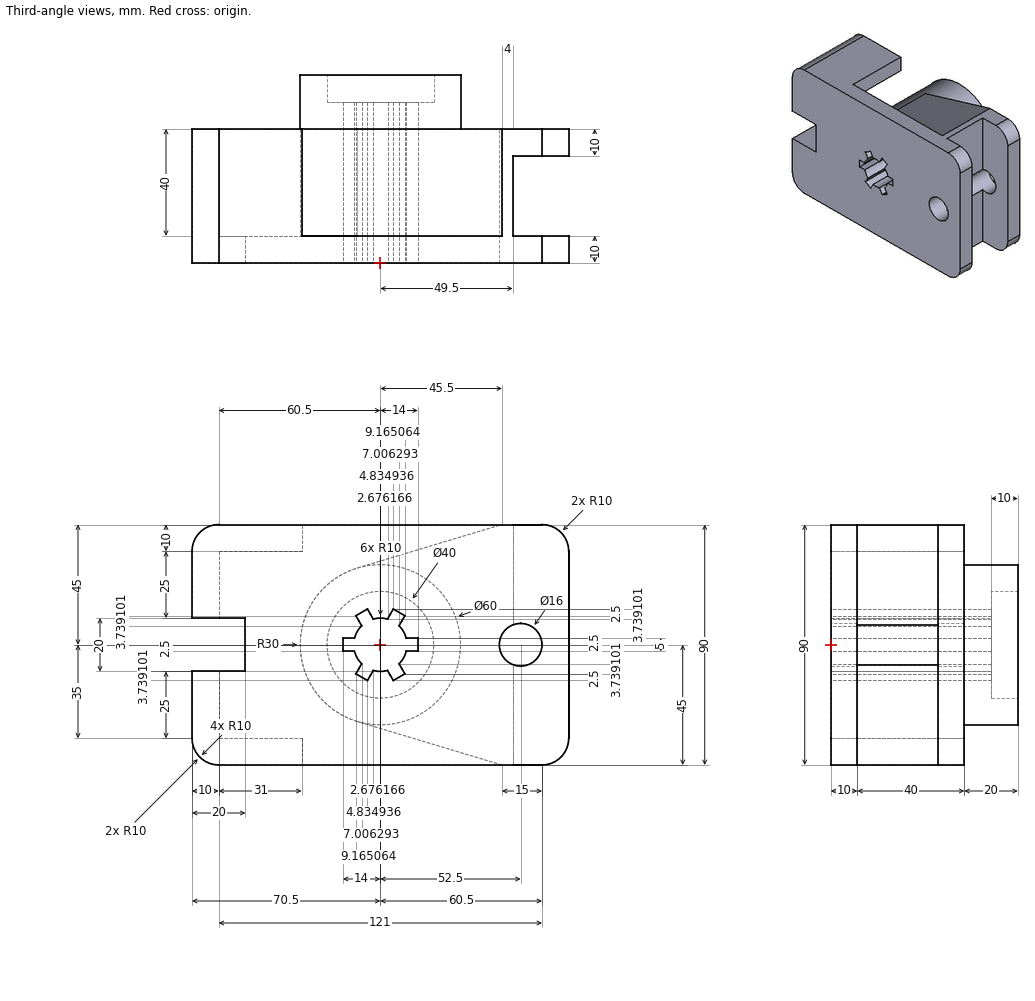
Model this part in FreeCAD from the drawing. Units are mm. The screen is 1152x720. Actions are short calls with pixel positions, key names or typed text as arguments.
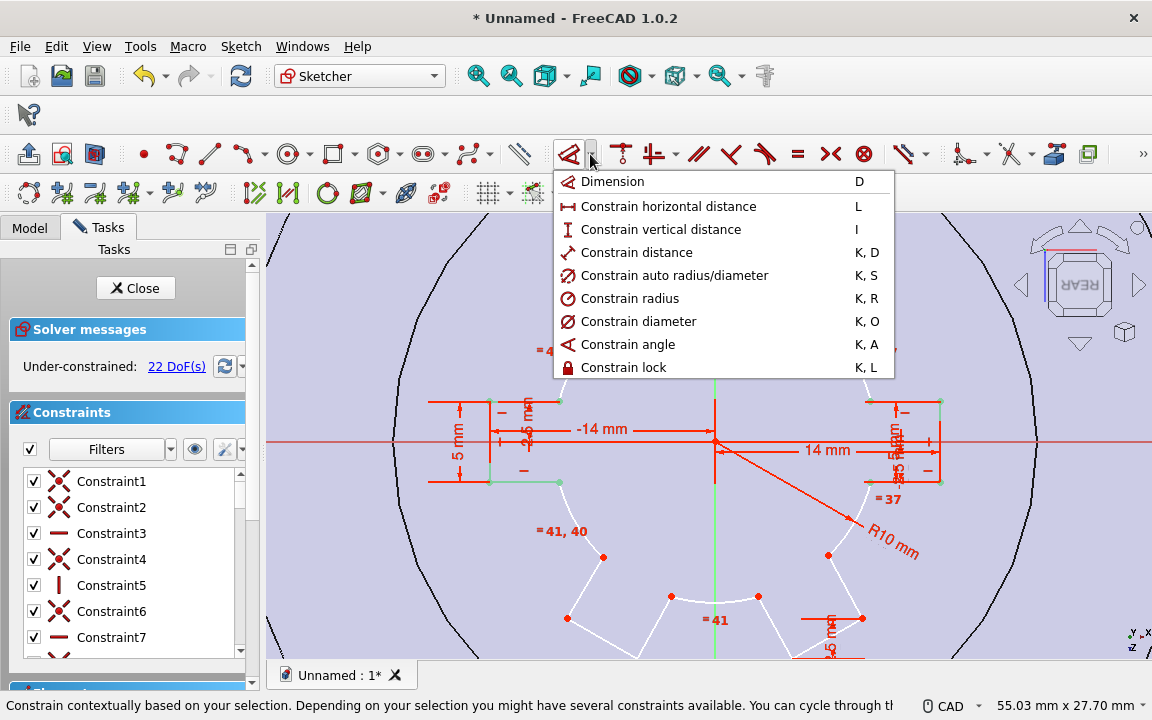
click(724, 230)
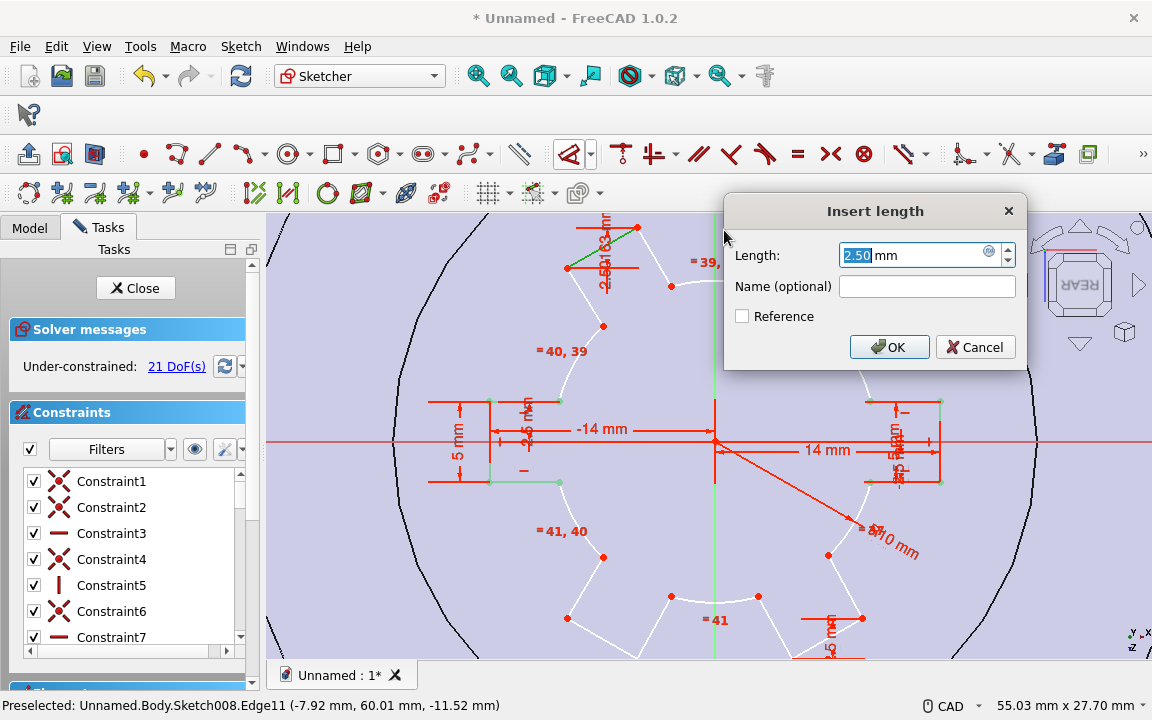
text(2.5)
key(Return)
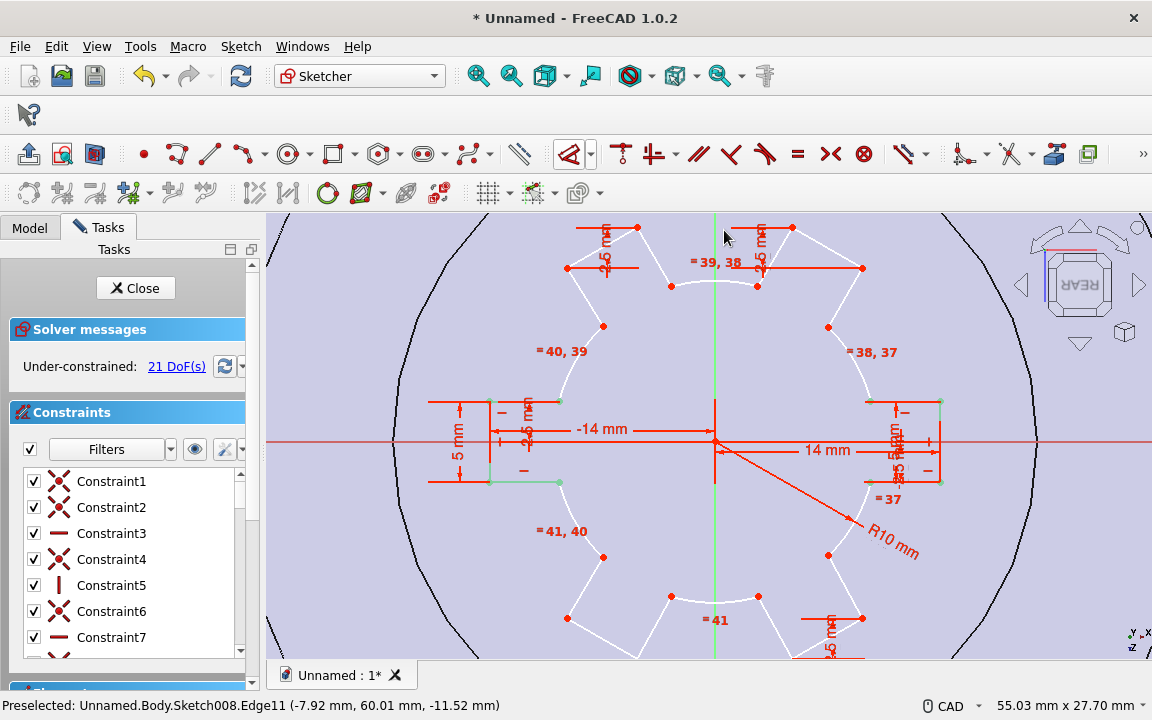
click(588, 631)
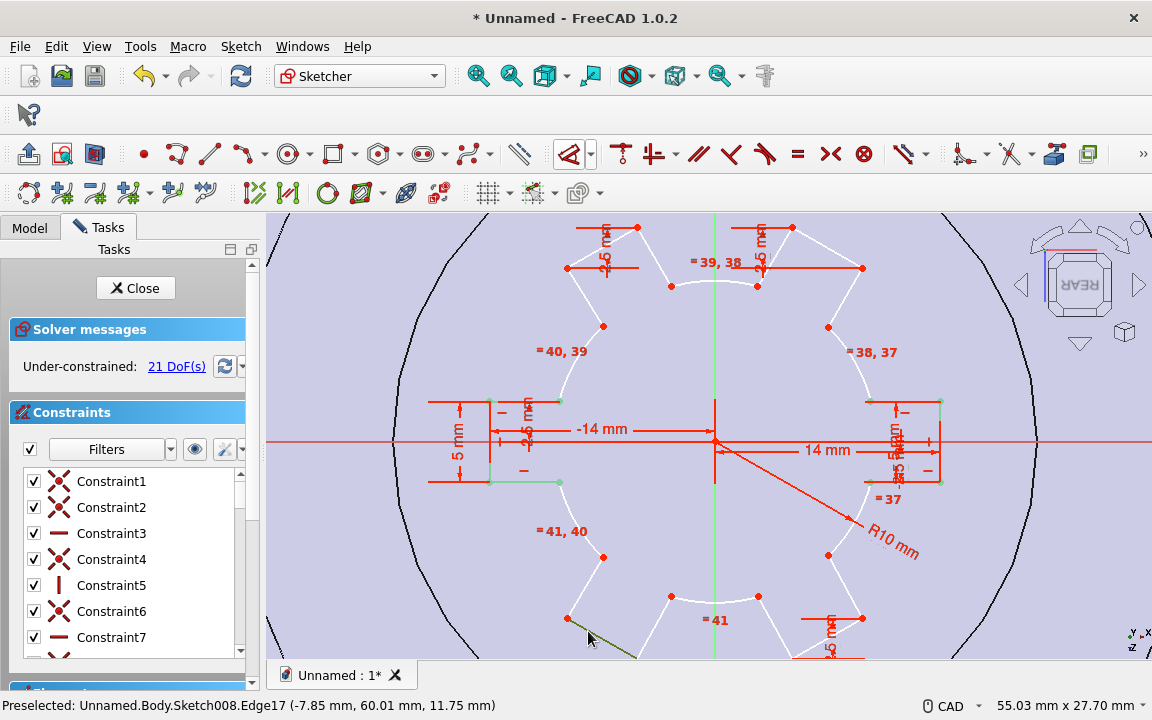
key(i)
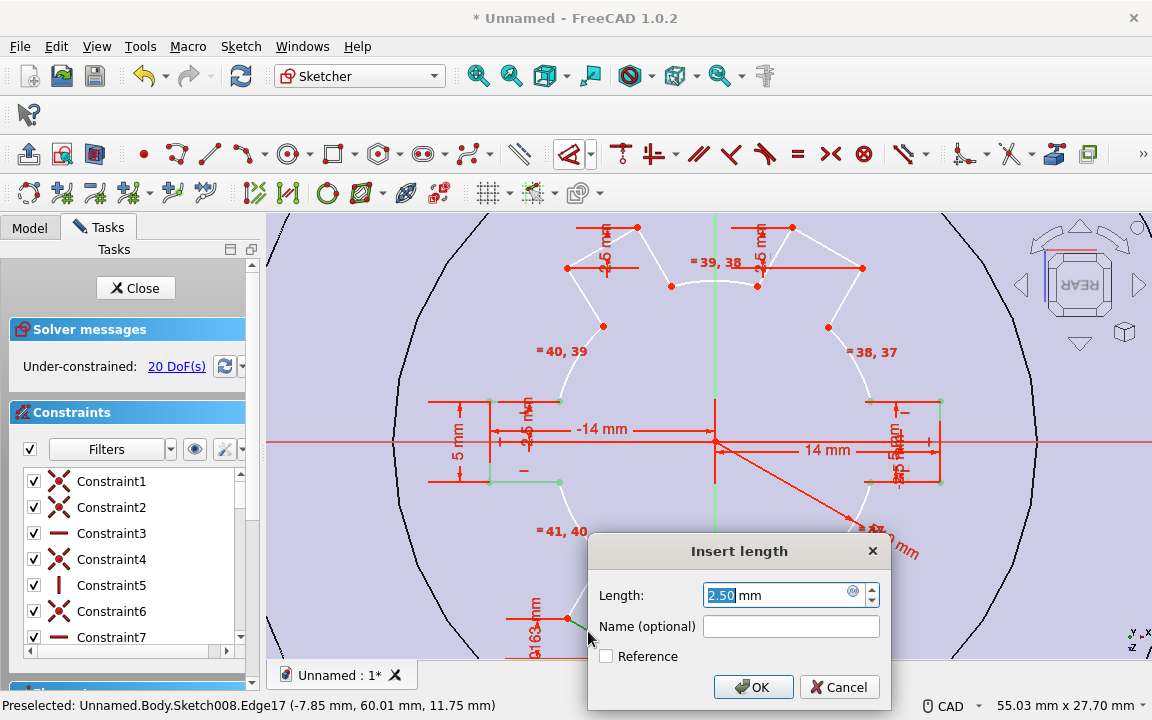
text(2.5)
key(Return)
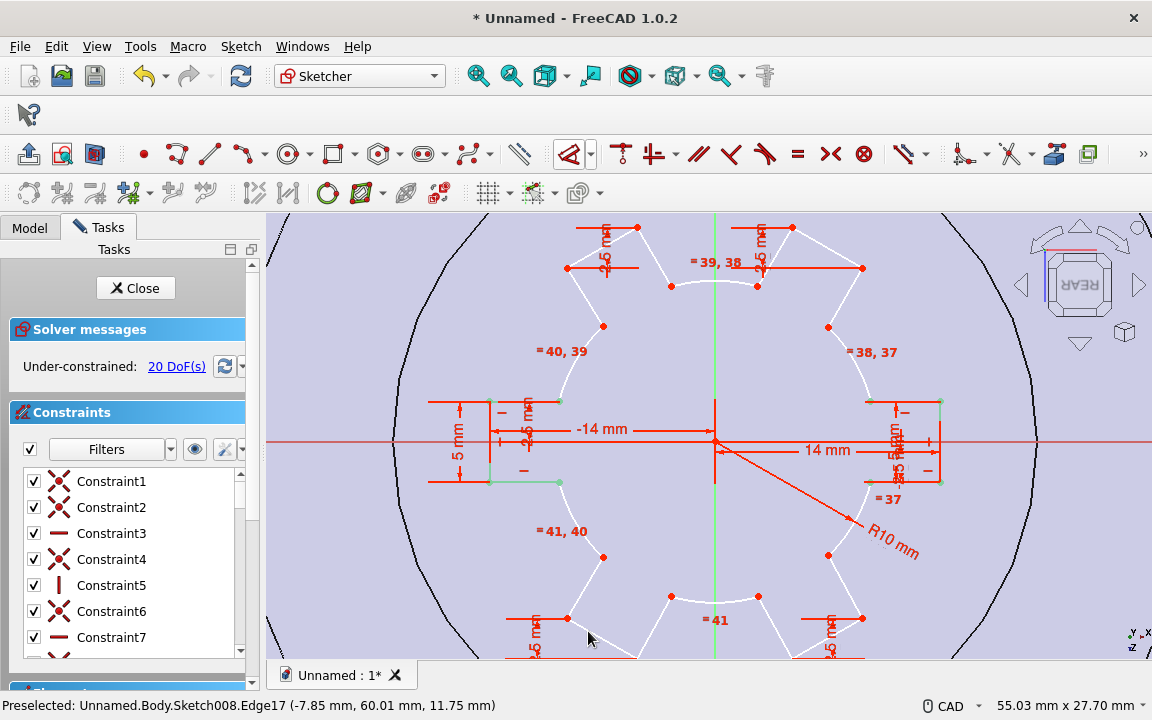
click(758, 597)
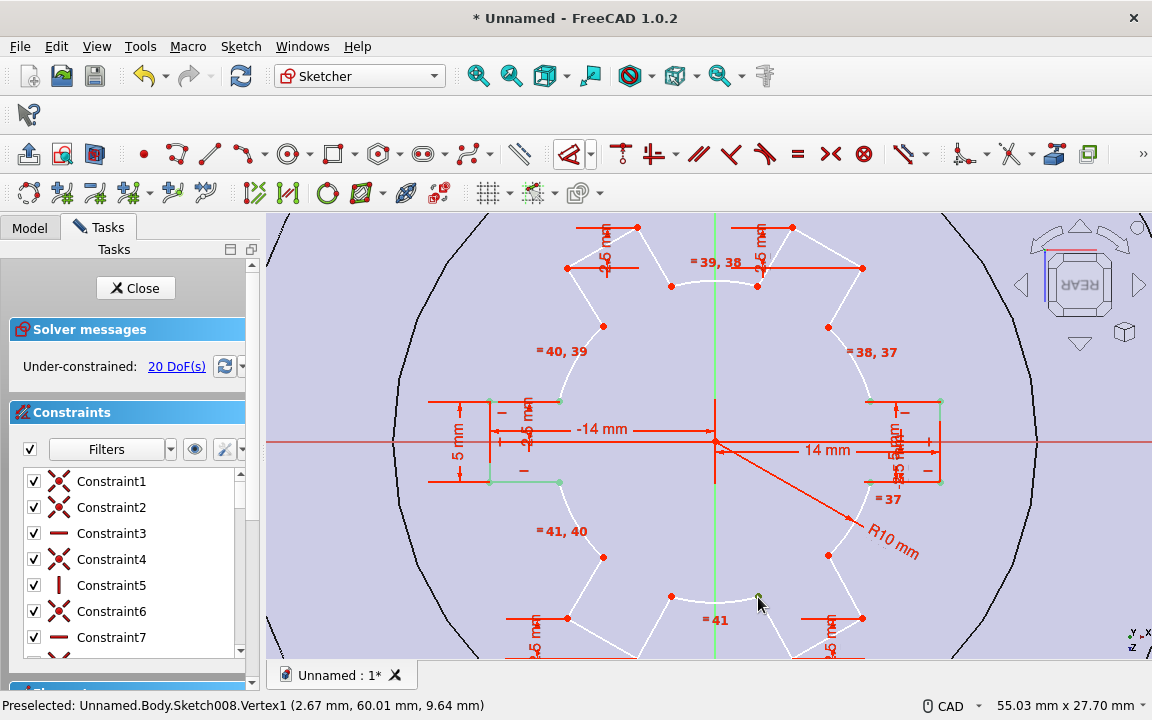
click(590, 154)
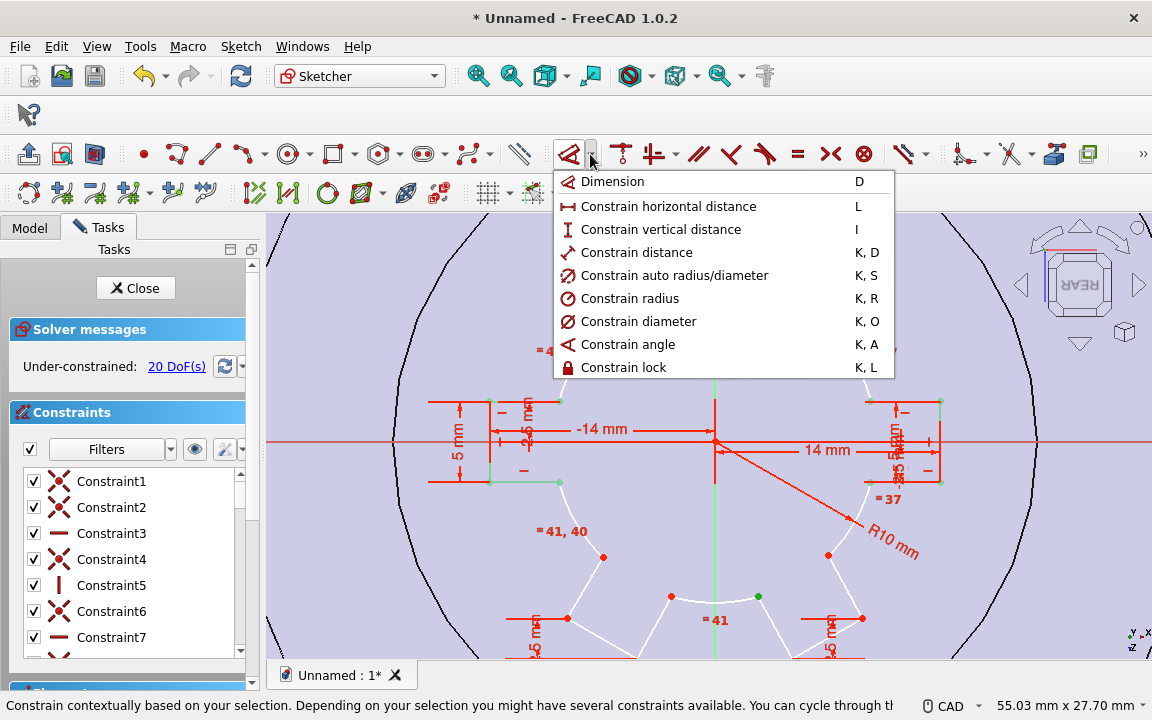
click(724, 206)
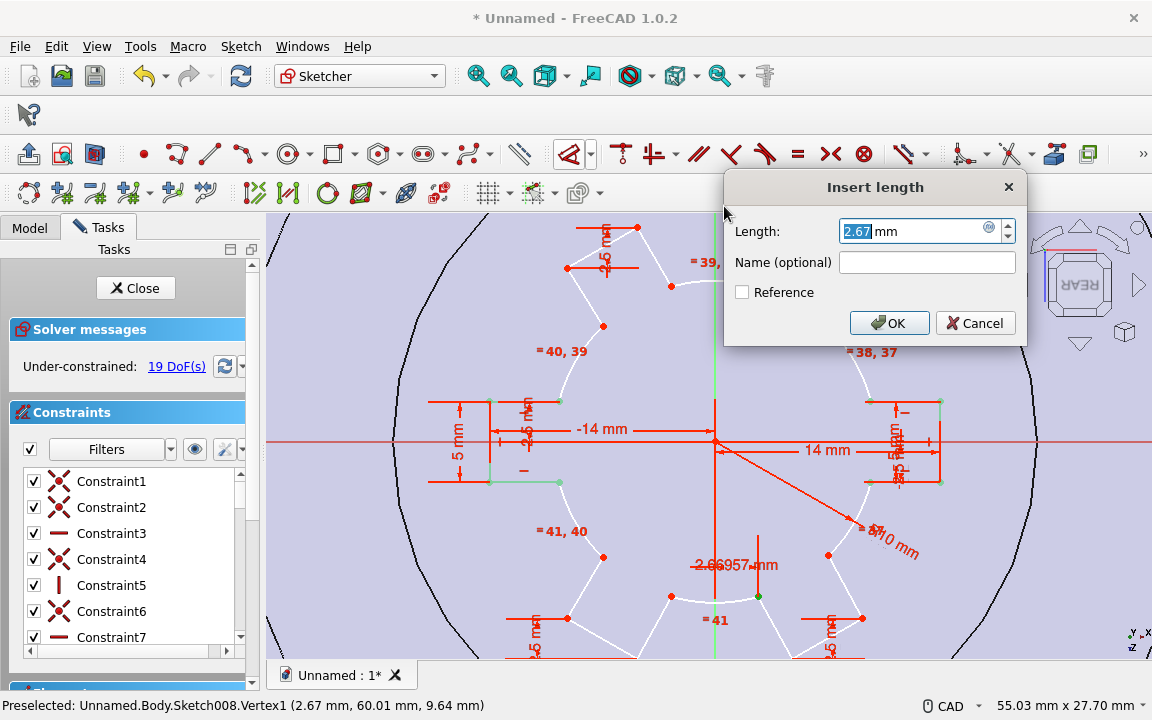
text(2.676166)
key(Return)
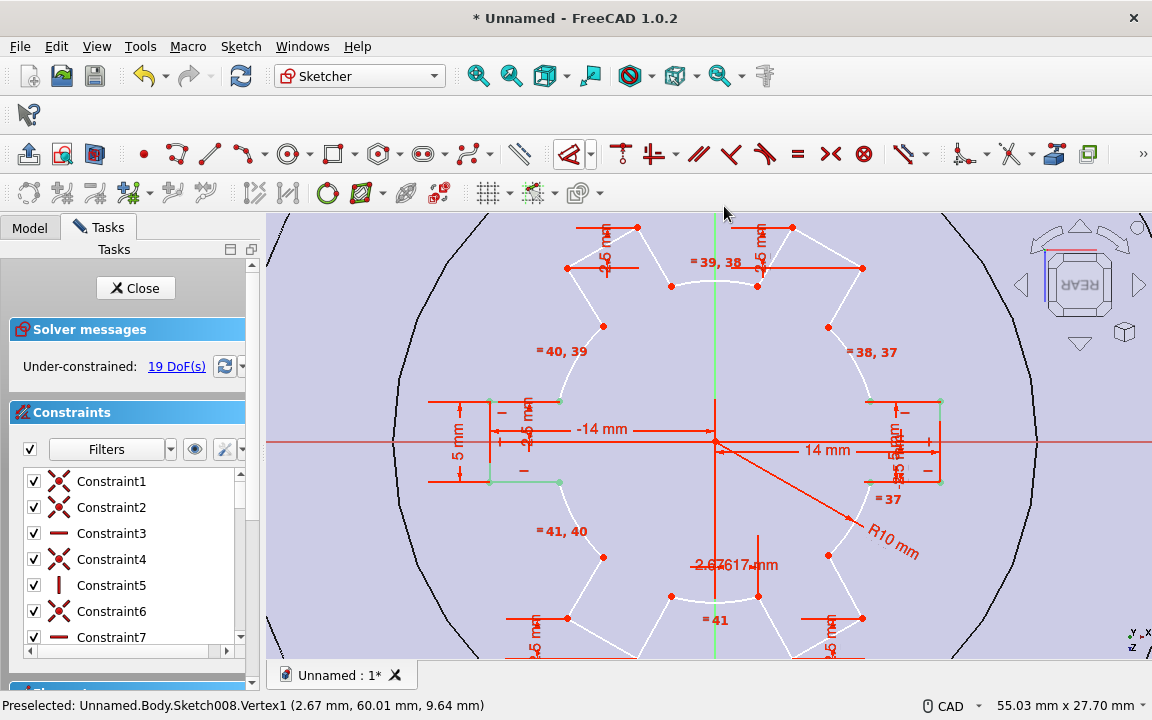
scroll(489, 424, down, 2)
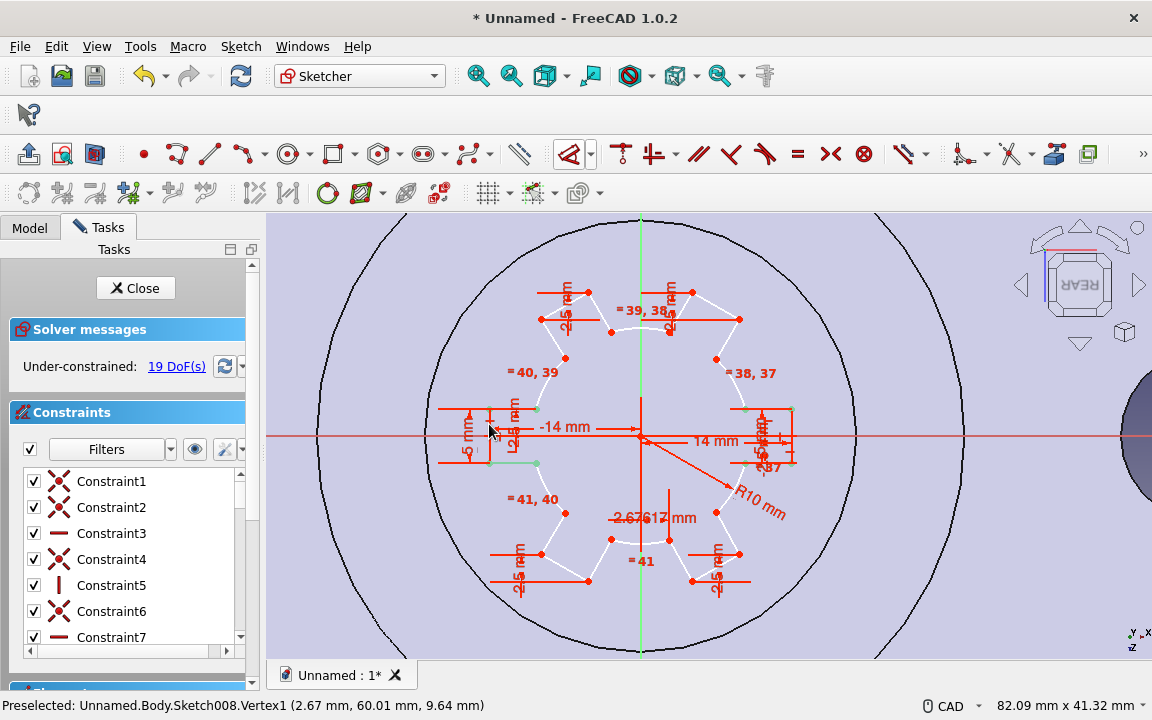
click(692, 582)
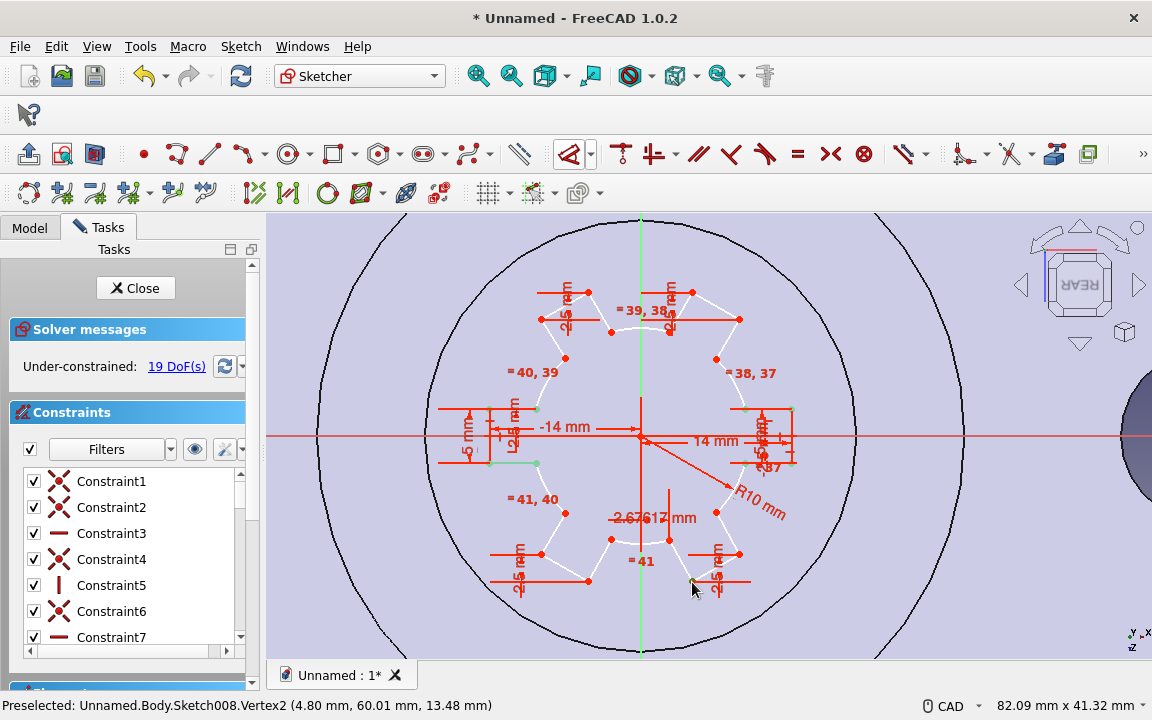
click(590, 154)